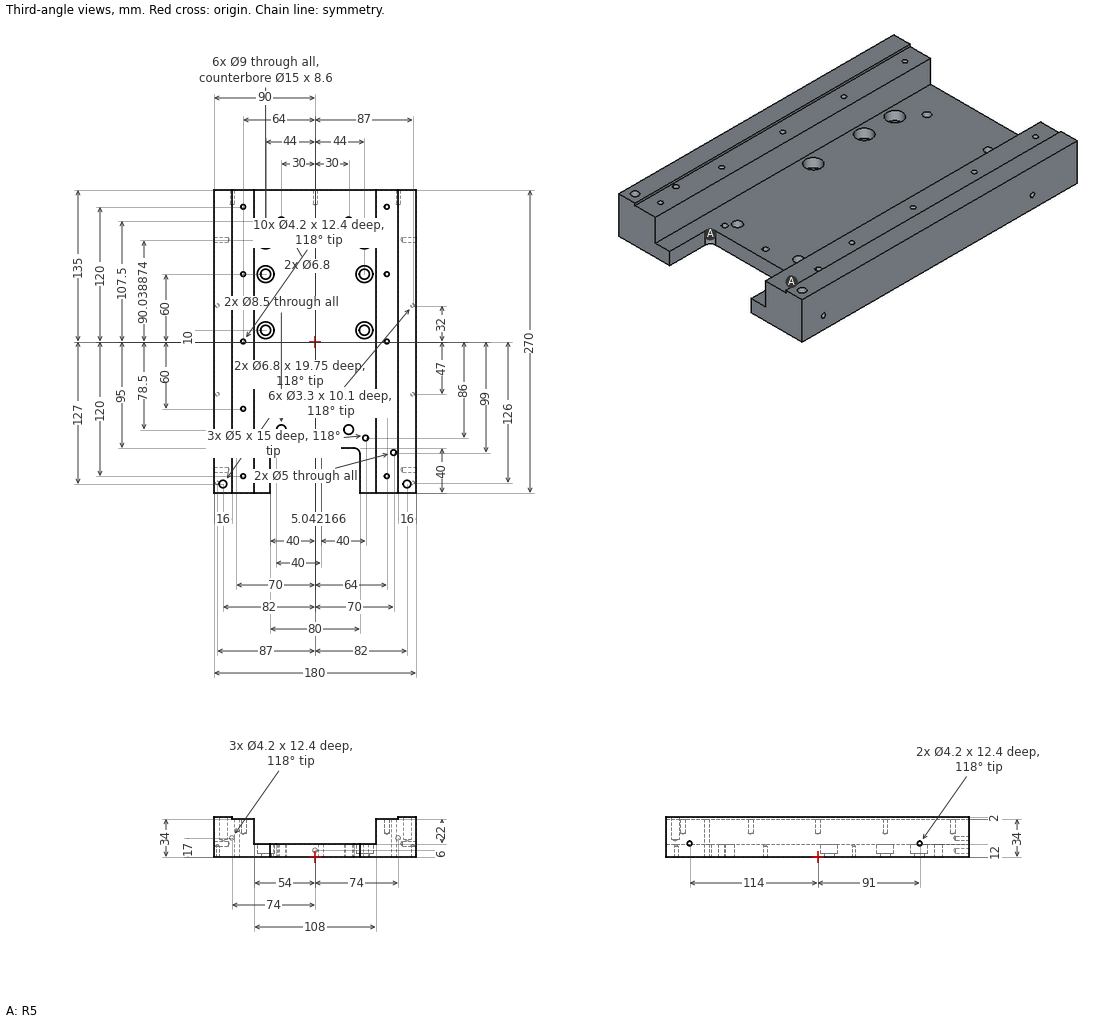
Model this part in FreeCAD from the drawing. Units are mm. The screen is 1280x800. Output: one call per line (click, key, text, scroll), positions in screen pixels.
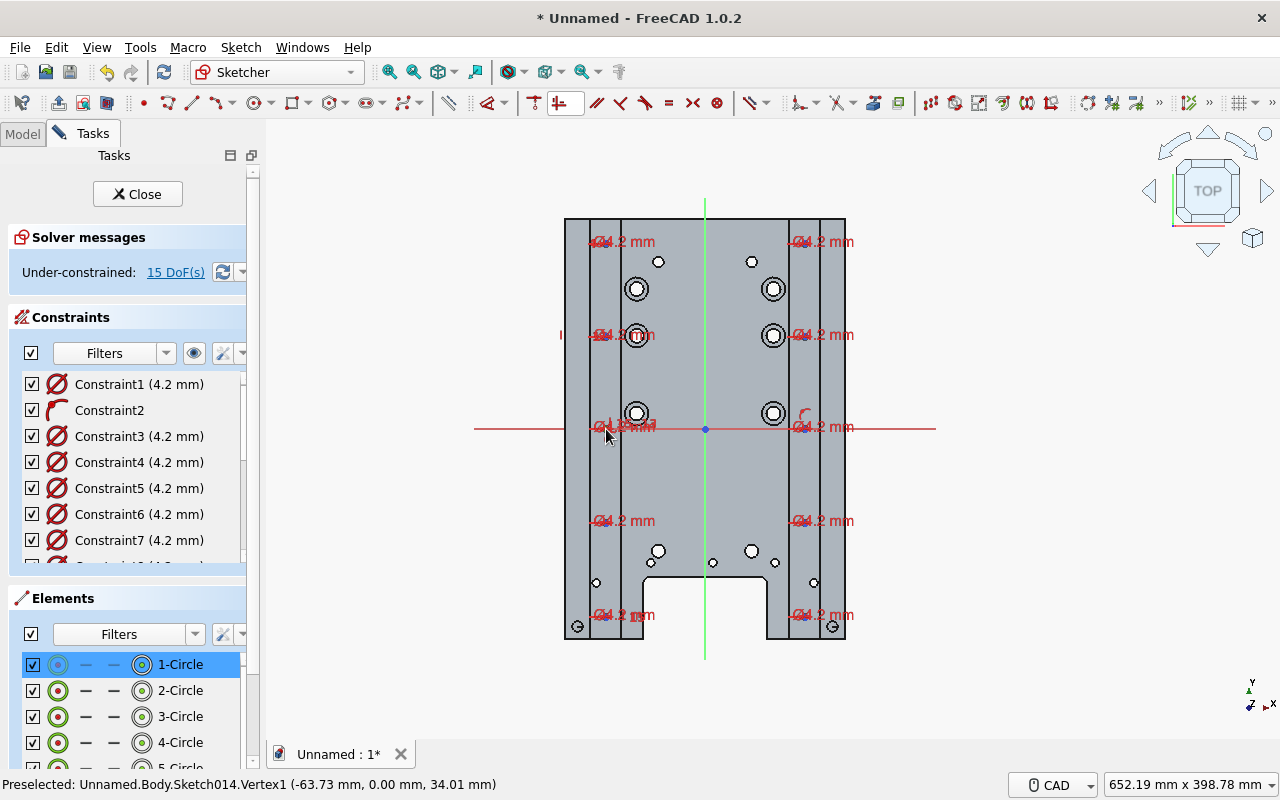
click(606, 523)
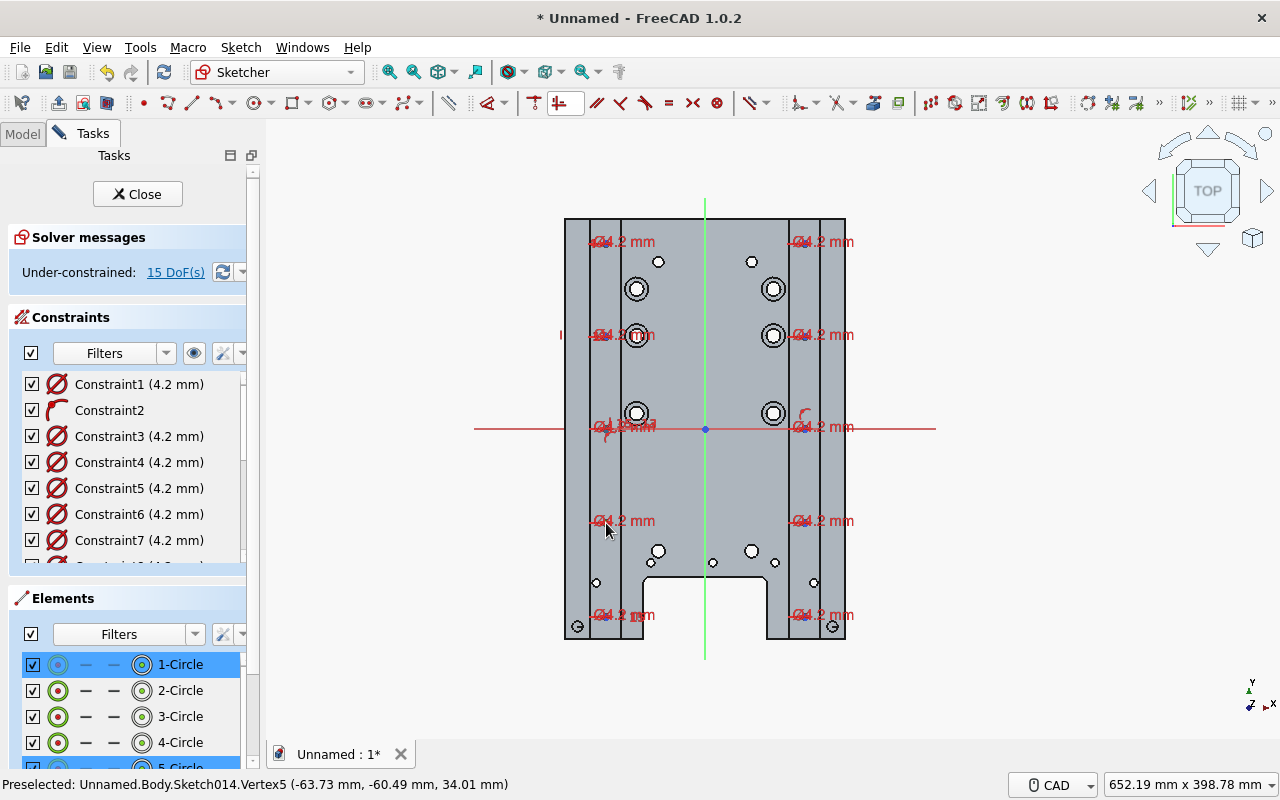
key(v)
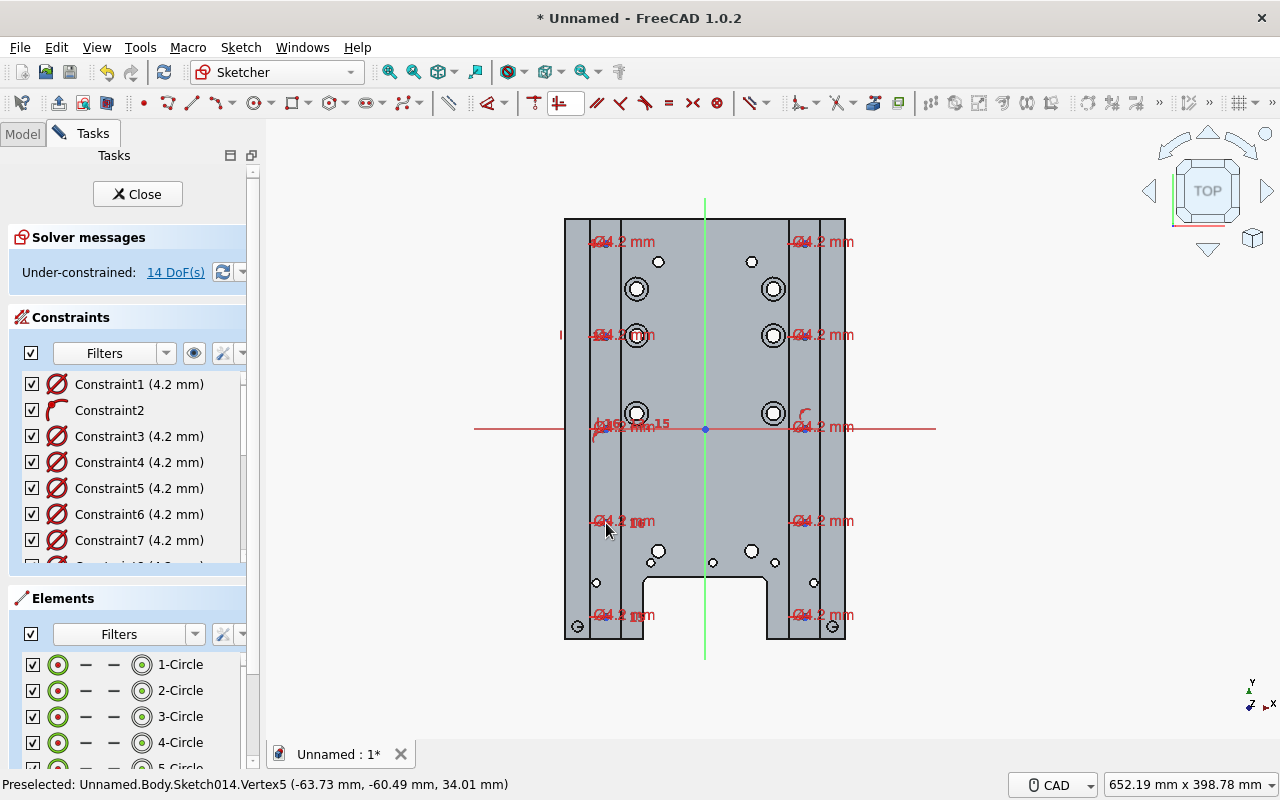
click(606, 523)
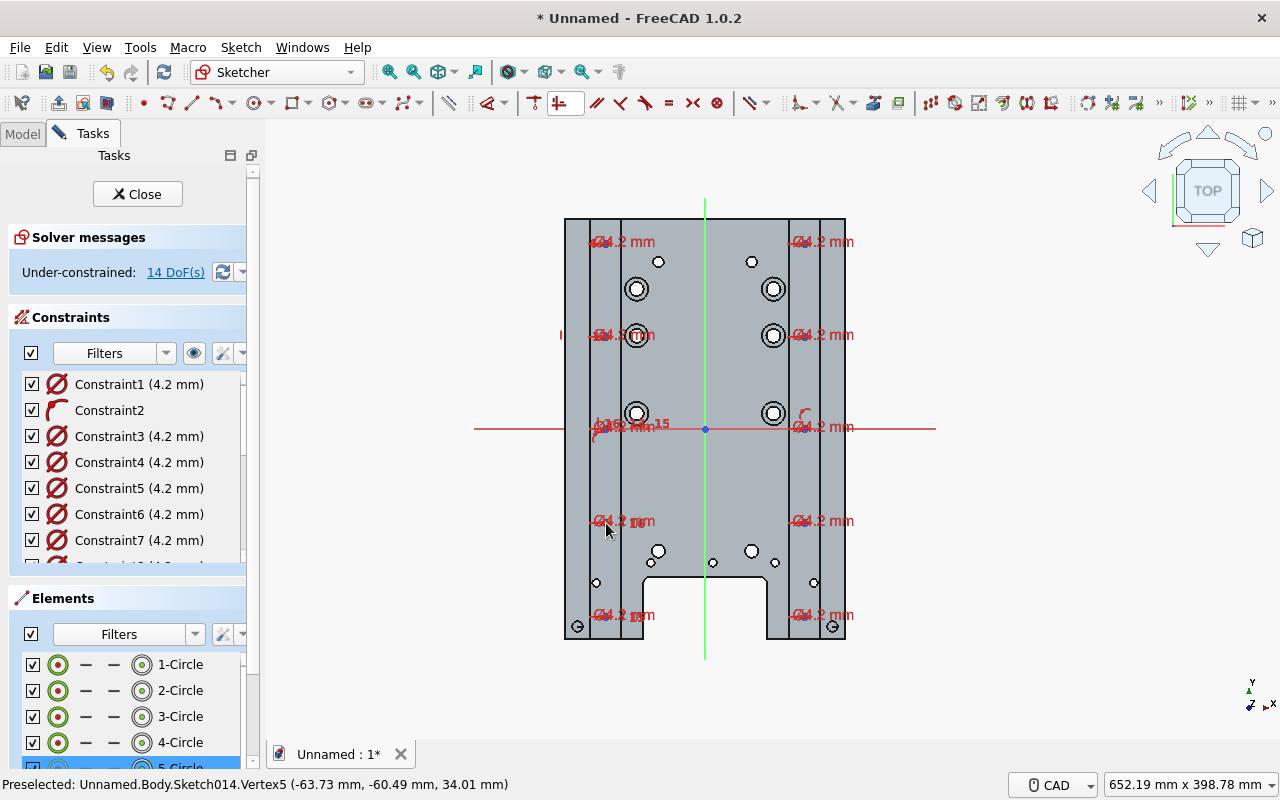
click(805, 523)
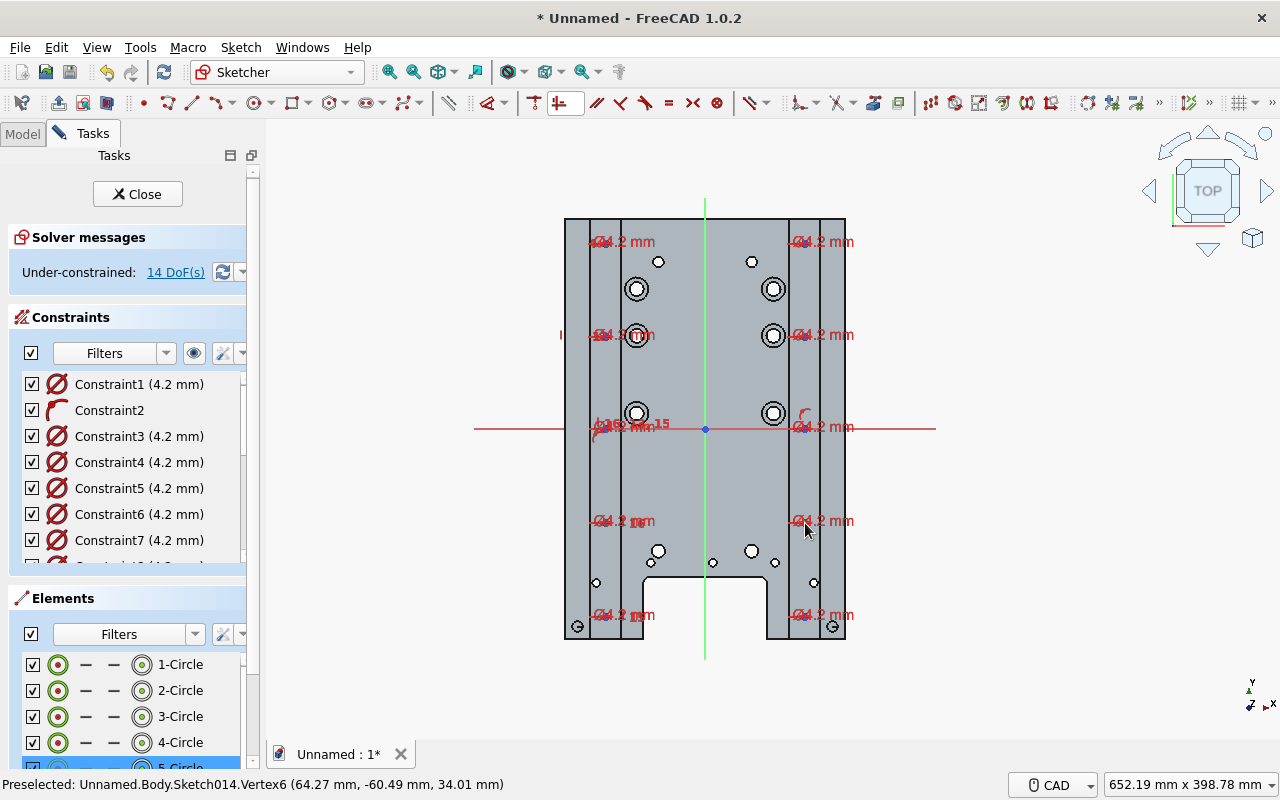
click(578, 104)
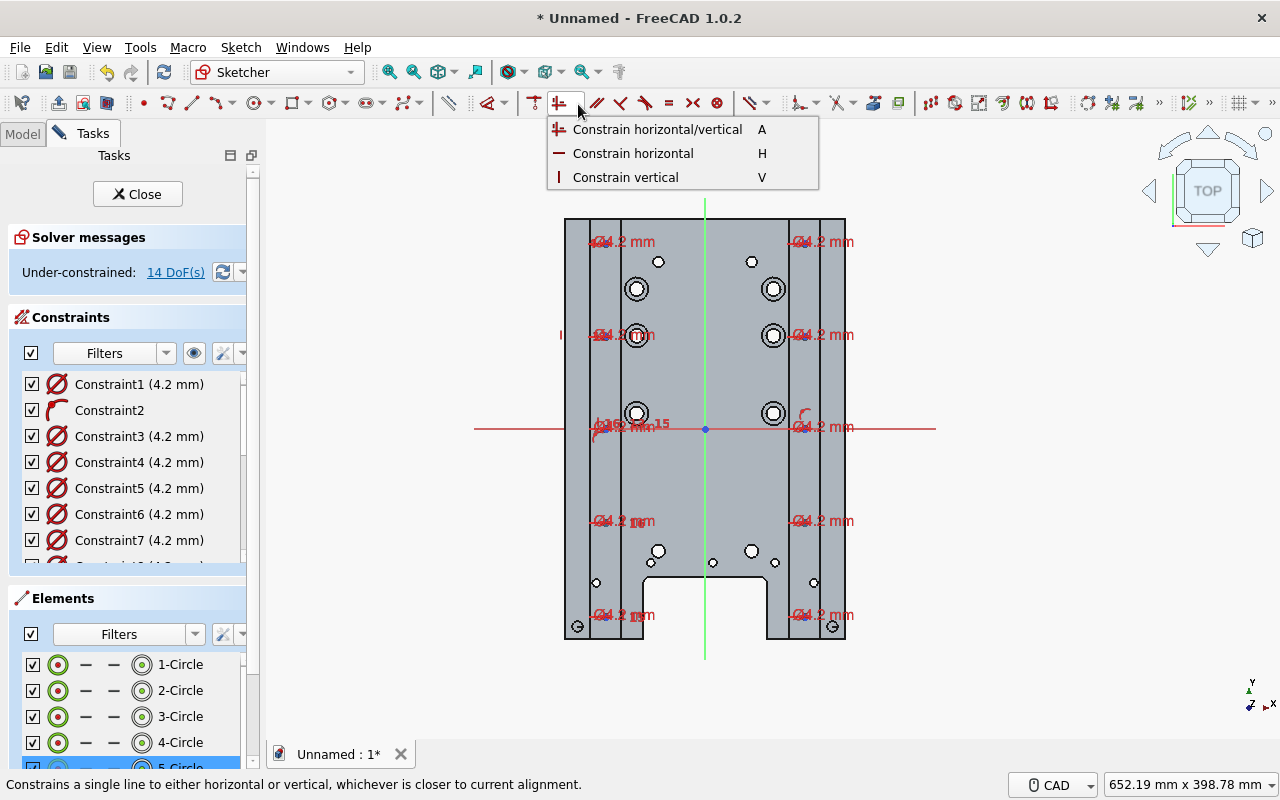
click(683, 153)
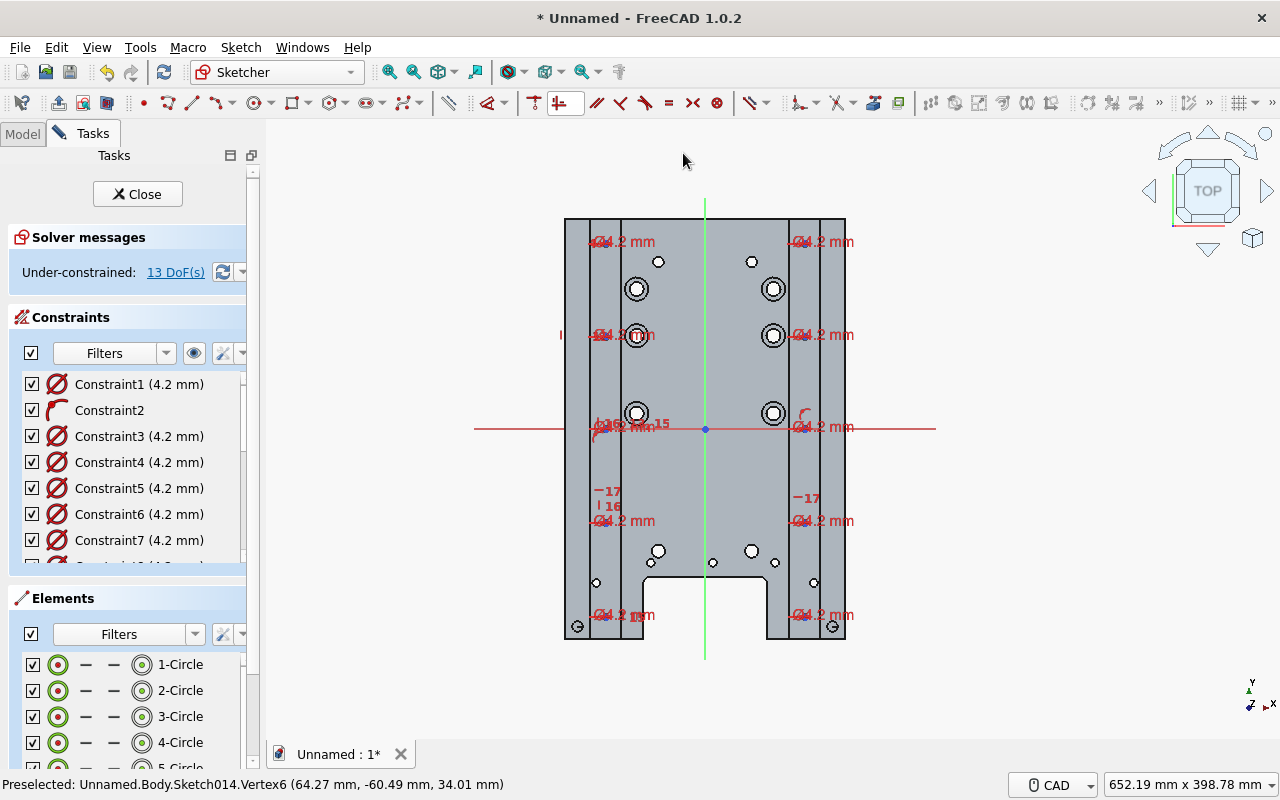
click(805, 523)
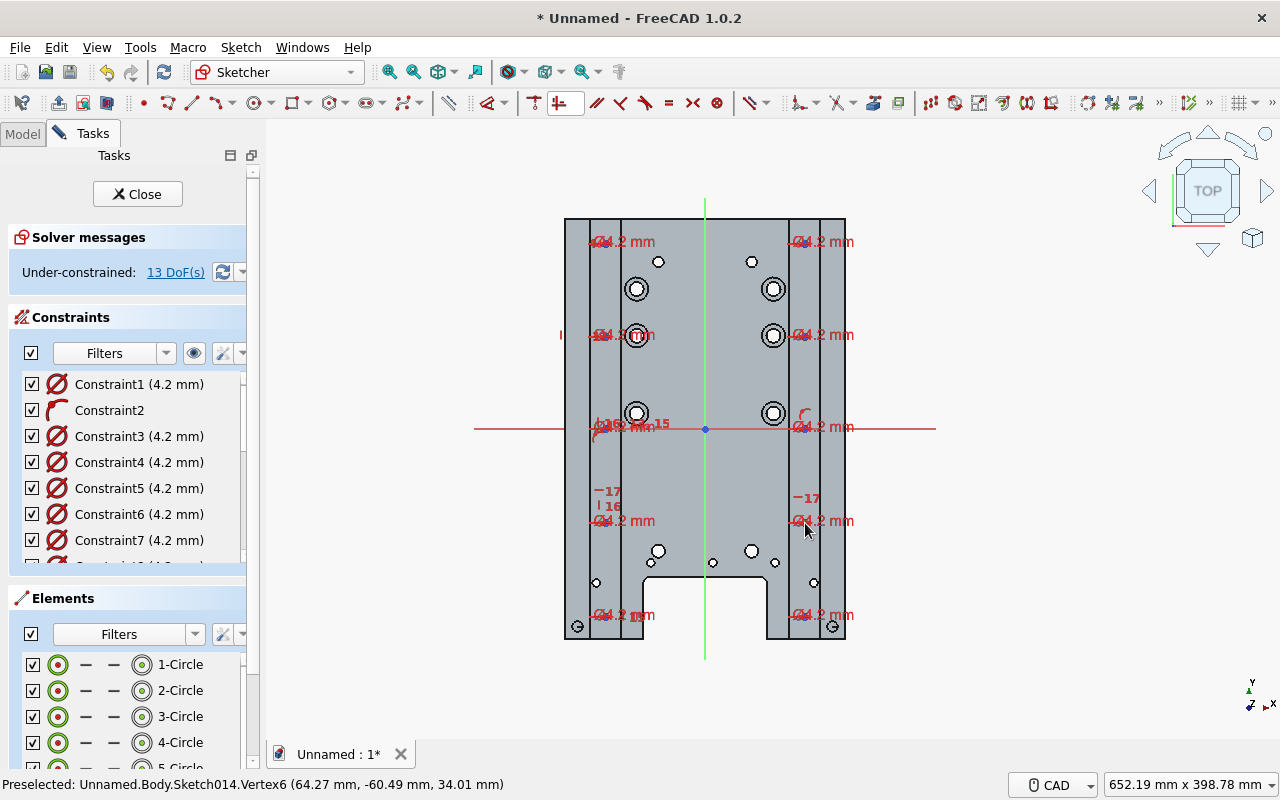
click(805, 617)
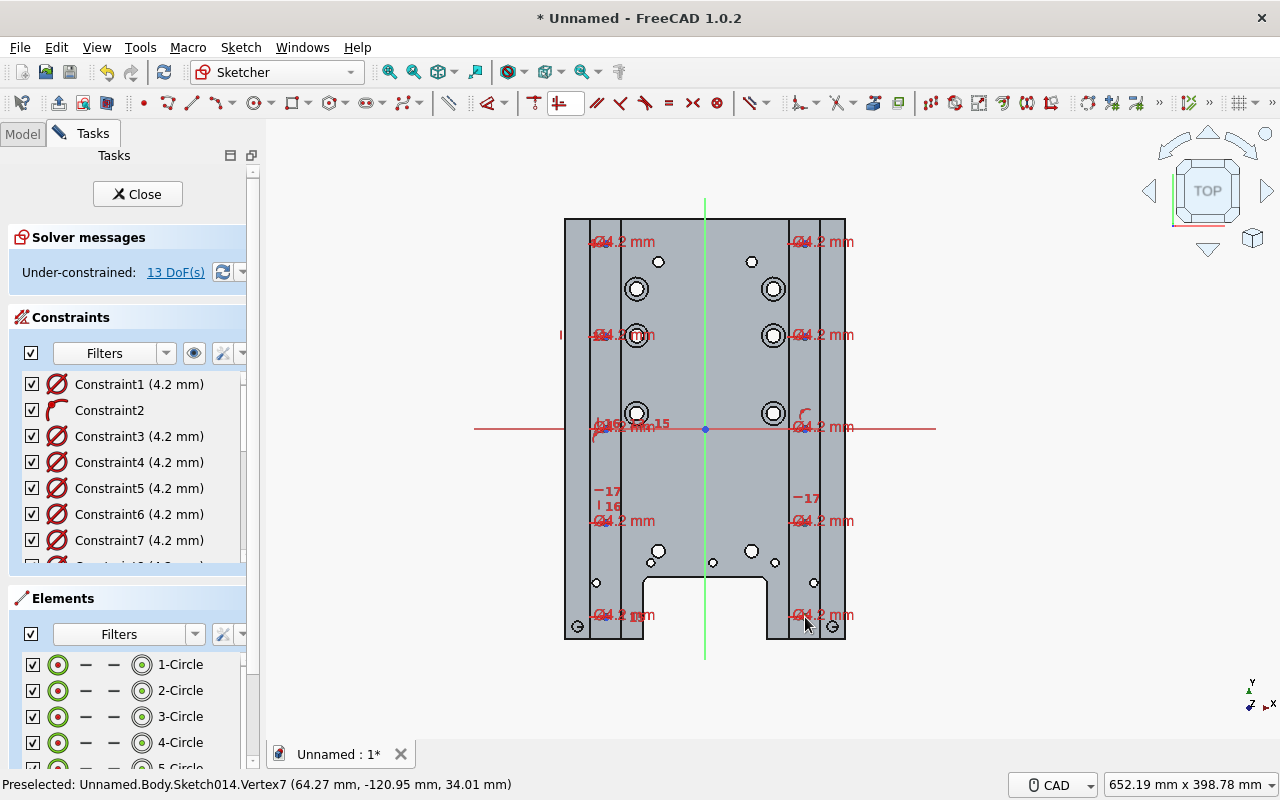
click(578, 104)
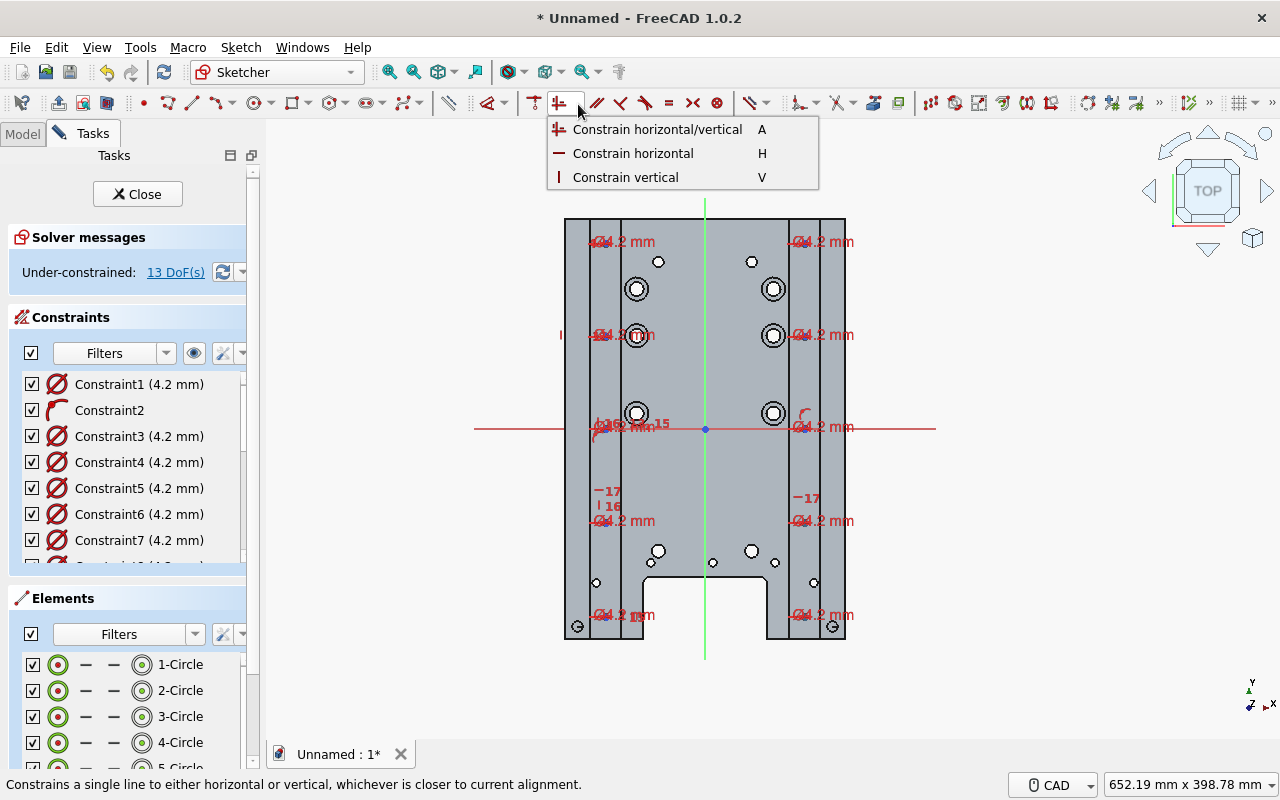
click(683, 177)